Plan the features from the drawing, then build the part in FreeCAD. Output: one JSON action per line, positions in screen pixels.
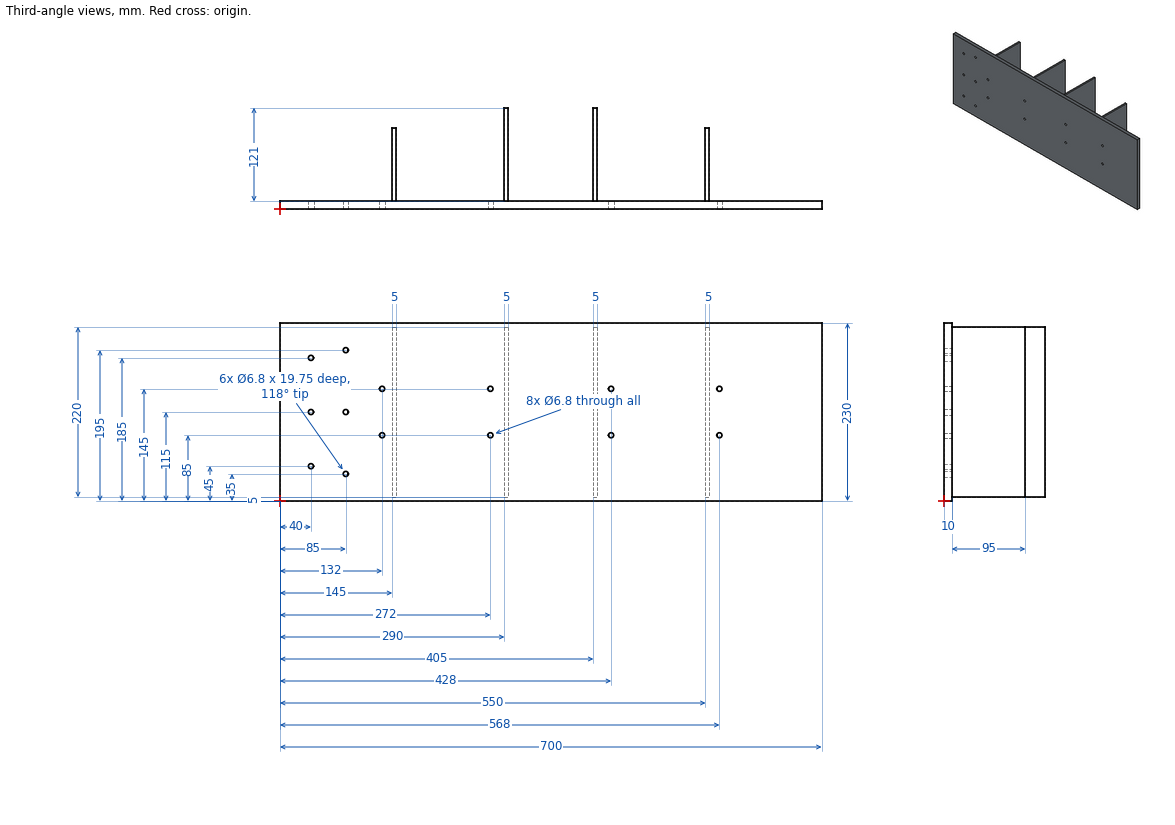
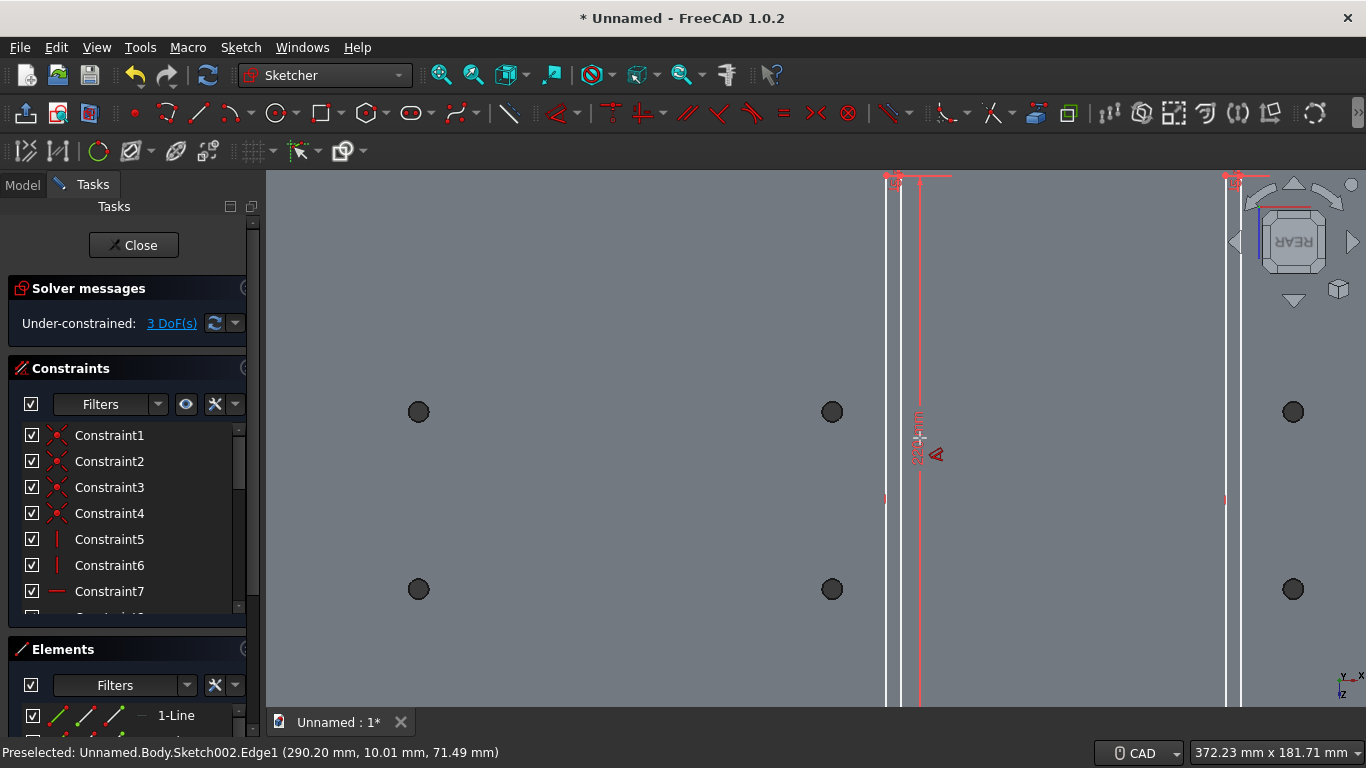
{"action": "scroll", "coordinate": [885, 372], "scroll_direction": "down", "scroll_amount": 3}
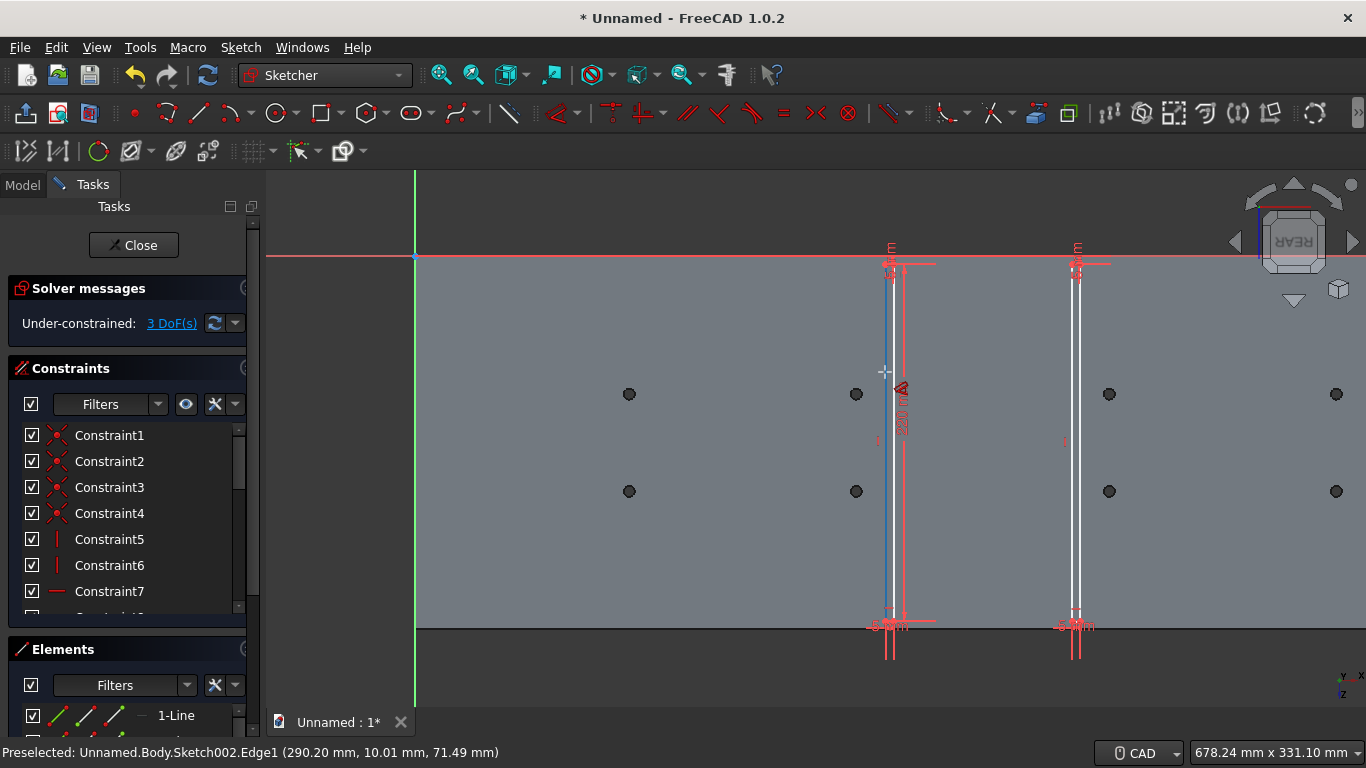
{"action": "scroll", "coordinate": [1072, 372], "scroll_direction": "up", "scroll_amount": 3}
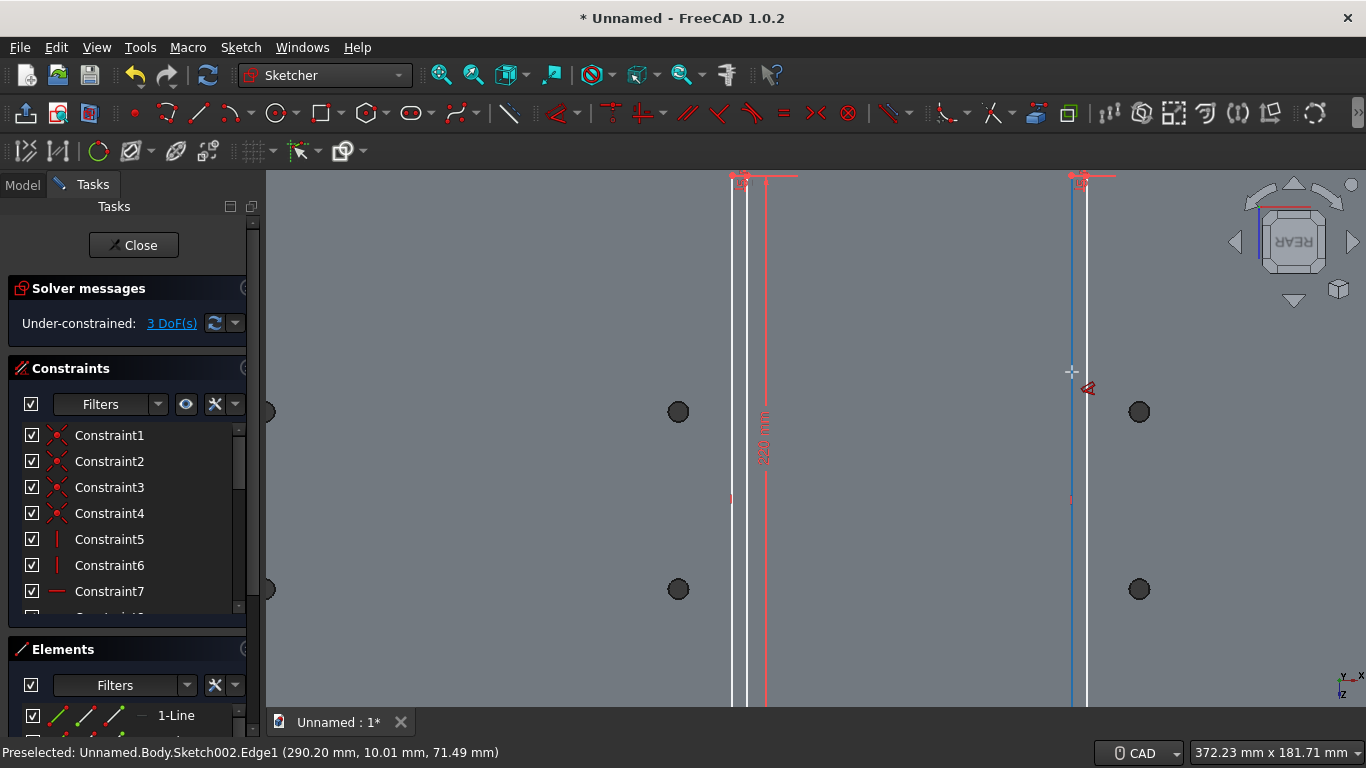
{"action": "left_click", "coordinate": [1072, 371]}
{"action": "left_click", "coordinate": [1106, 438]}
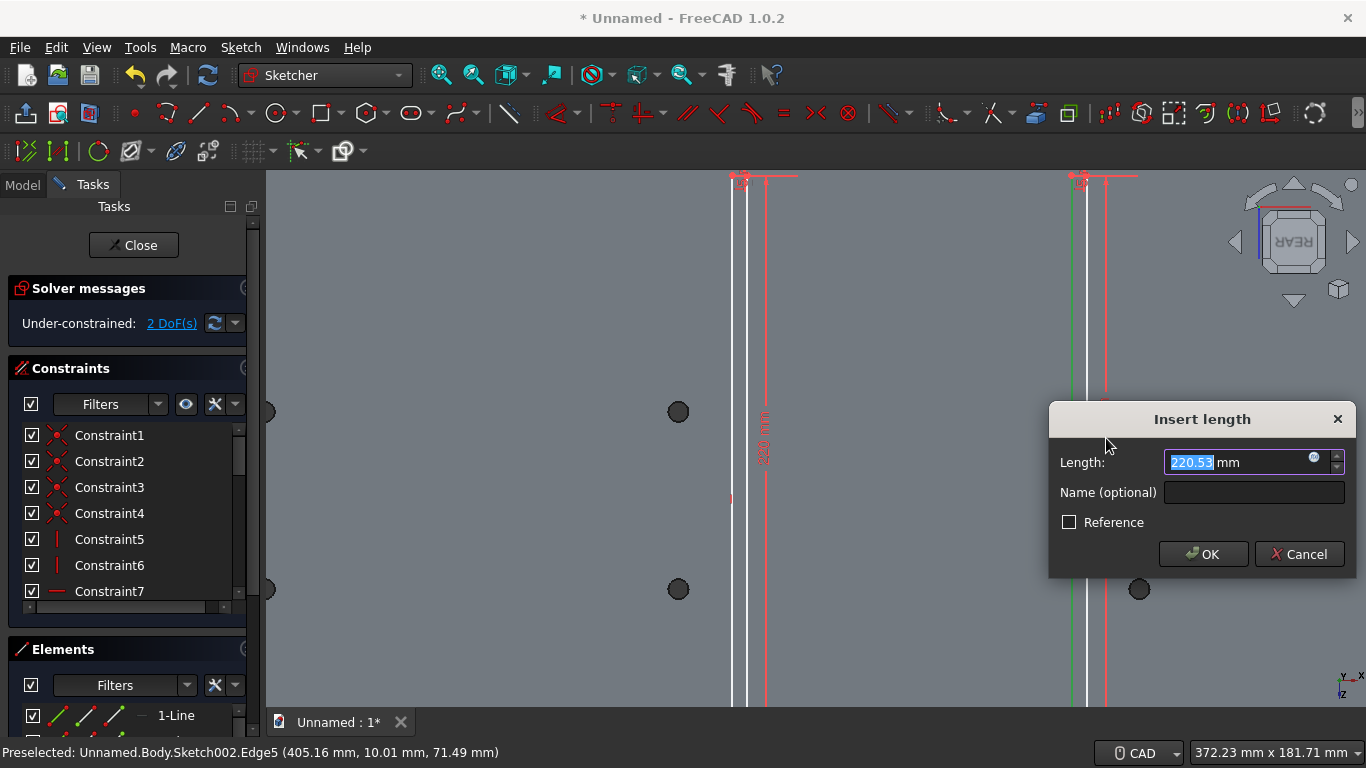
{"action": "type", "text": "220"}
{"action": "key", "text": "Return"}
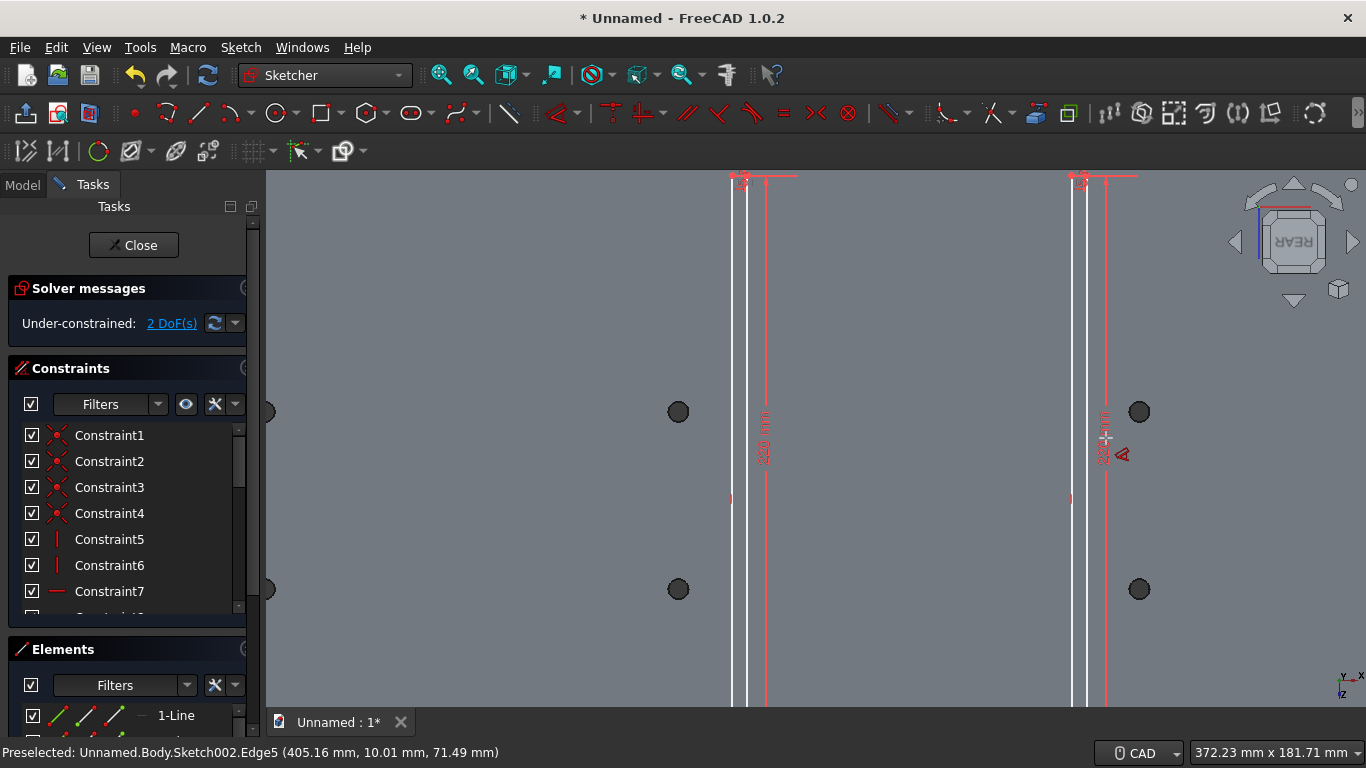
{"action": "scroll", "coordinate": [1072, 372], "scroll_direction": "down", "scroll_amount": 3}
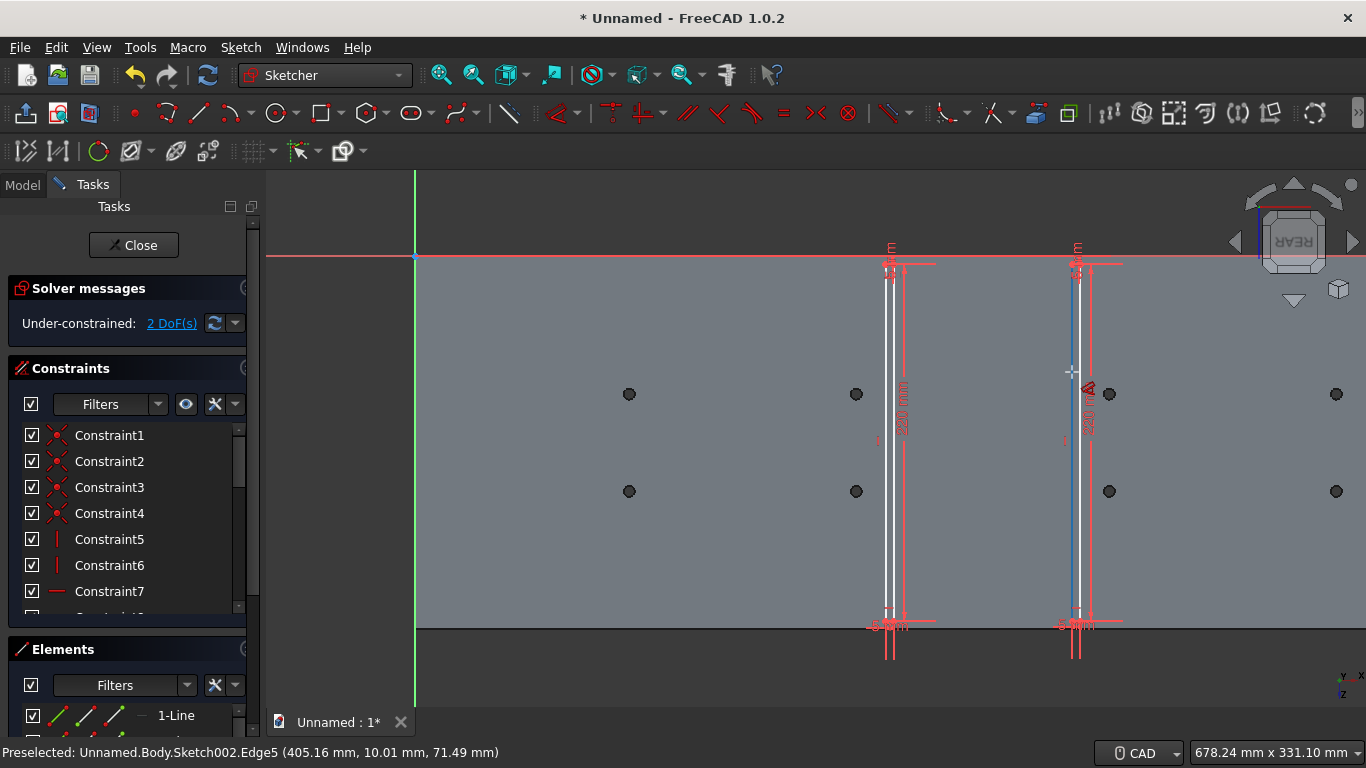
{"action": "scroll", "coordinate": [886, 264], "scroll_direction": "up", "scroll_amount": 3}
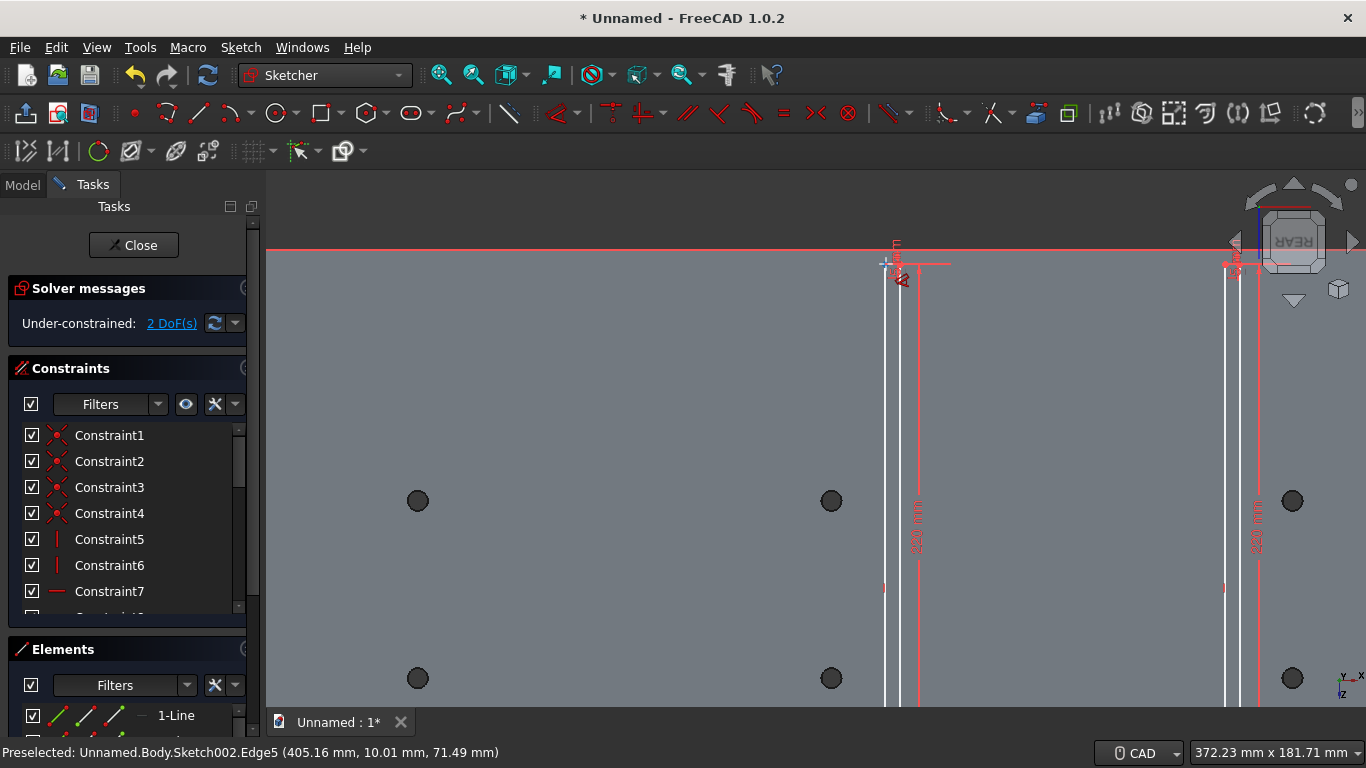
{"action": "left_click", "coordinate": [885, 264]}
{"action": "left_click", "coordinate": [590, 216]}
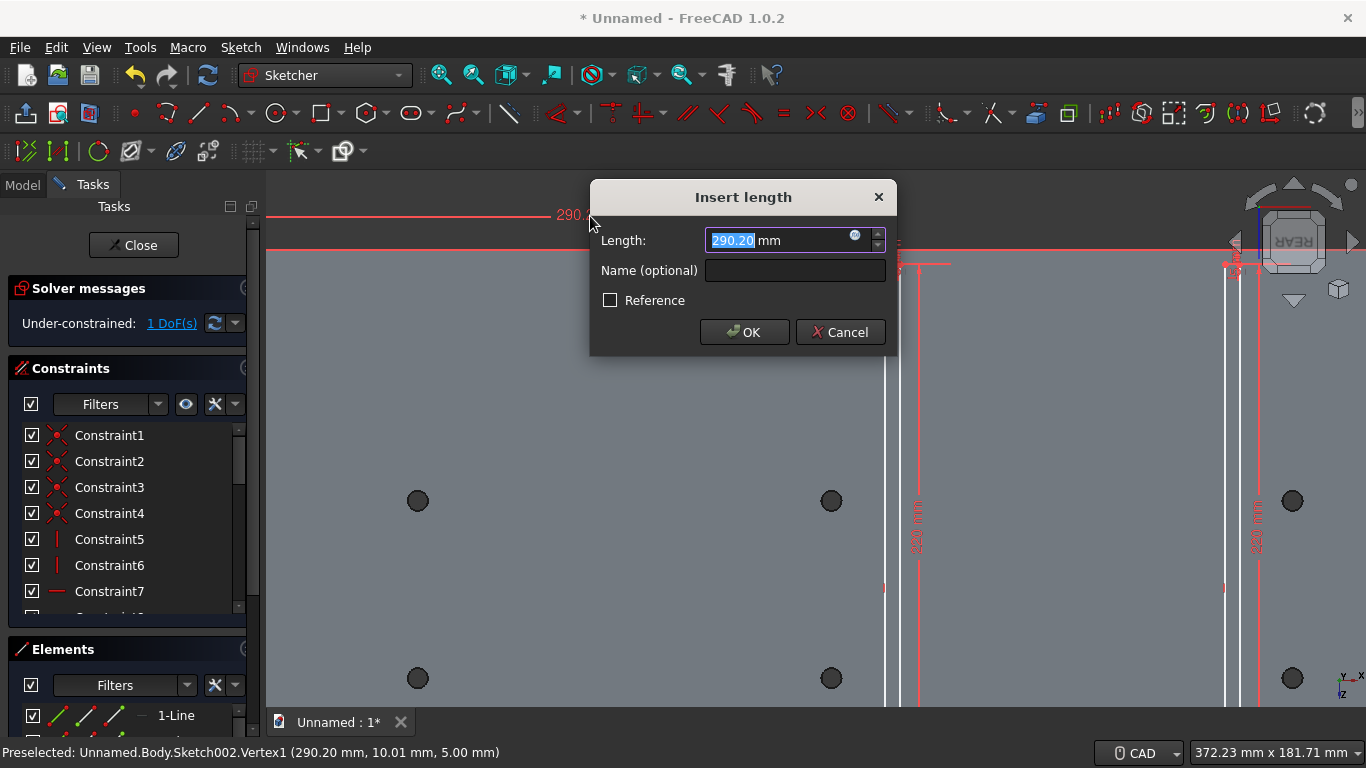
{"action": "type", "text": "290"}
{"action": "key", "text": "Return"}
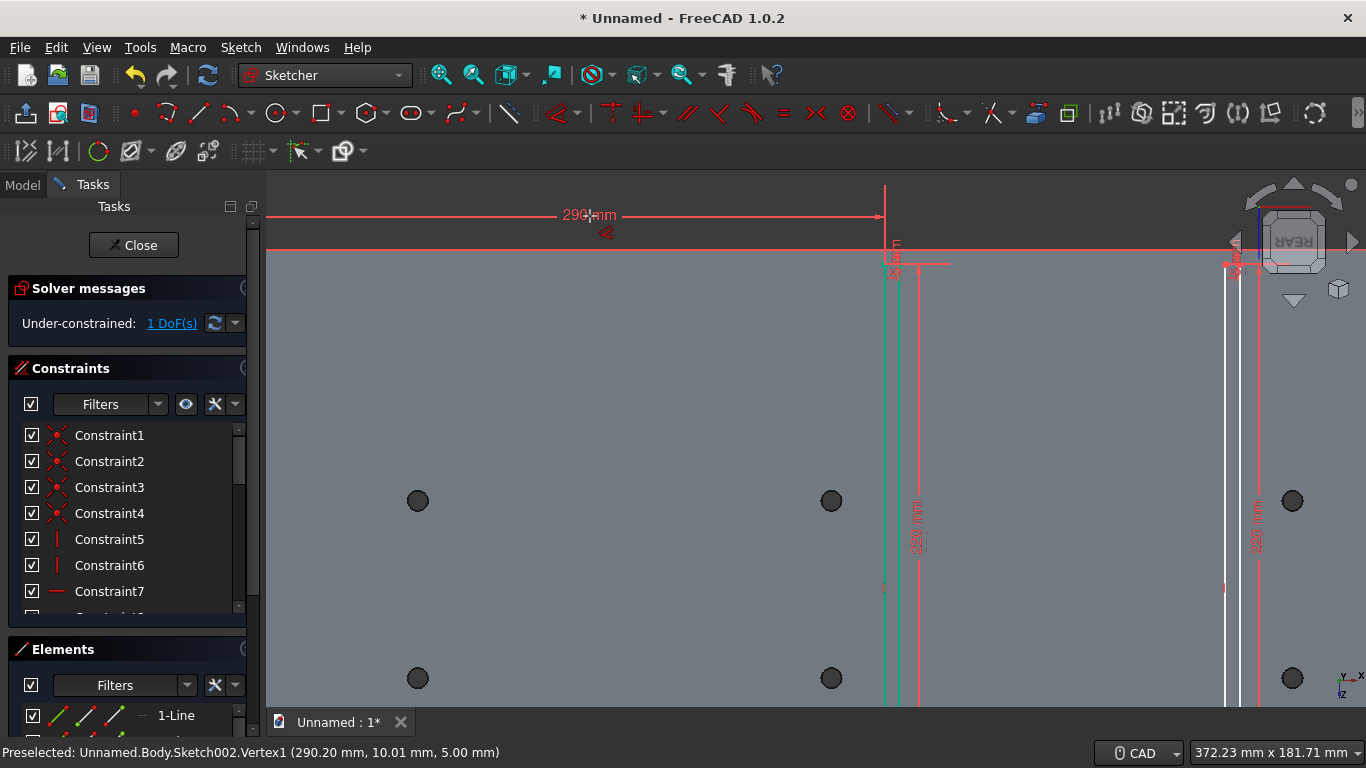
{"action": "scroll", "coordinate": [886, 264], "scroll_direction": "down", "scroll_amount": 3}